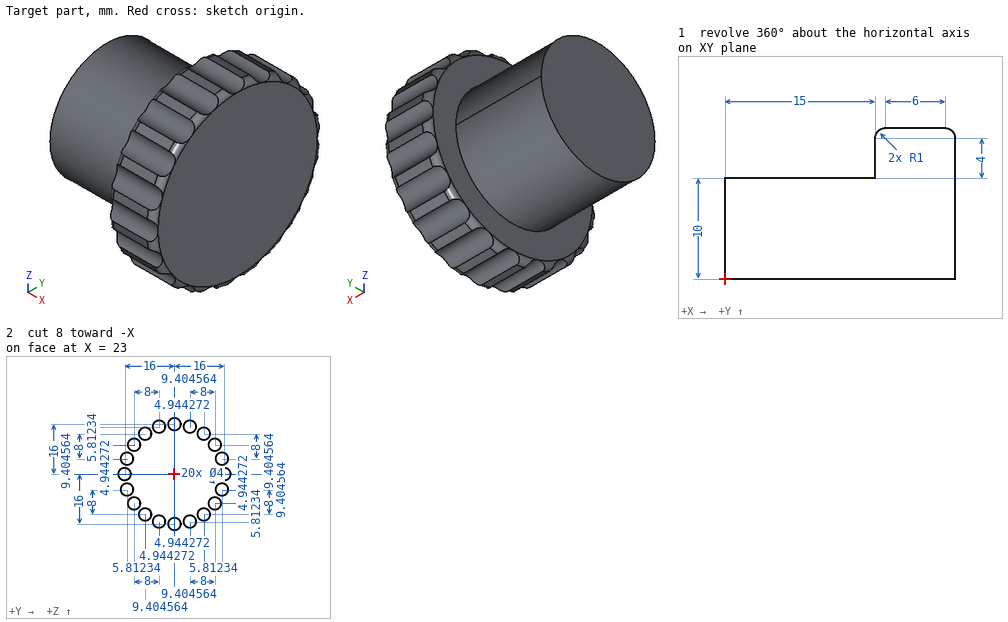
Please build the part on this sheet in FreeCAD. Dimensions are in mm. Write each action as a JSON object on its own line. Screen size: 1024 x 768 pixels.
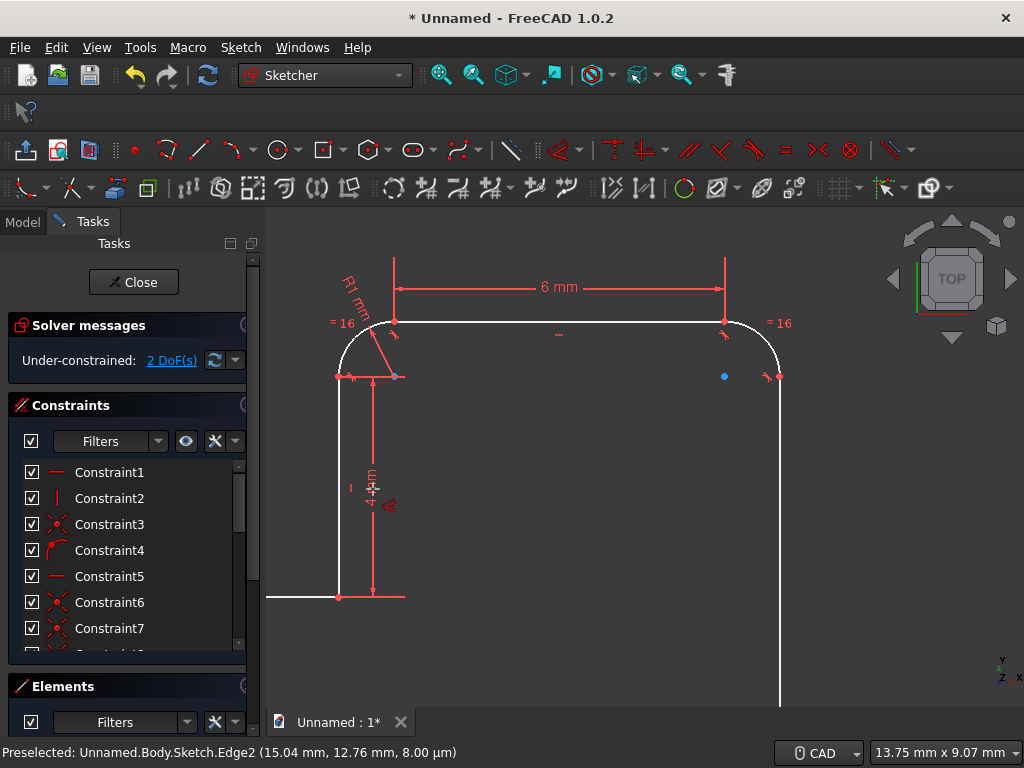
{"action": "scroll", "coordinate": [763, 337], "scroll_direction": "down", "scroll_amount": 6}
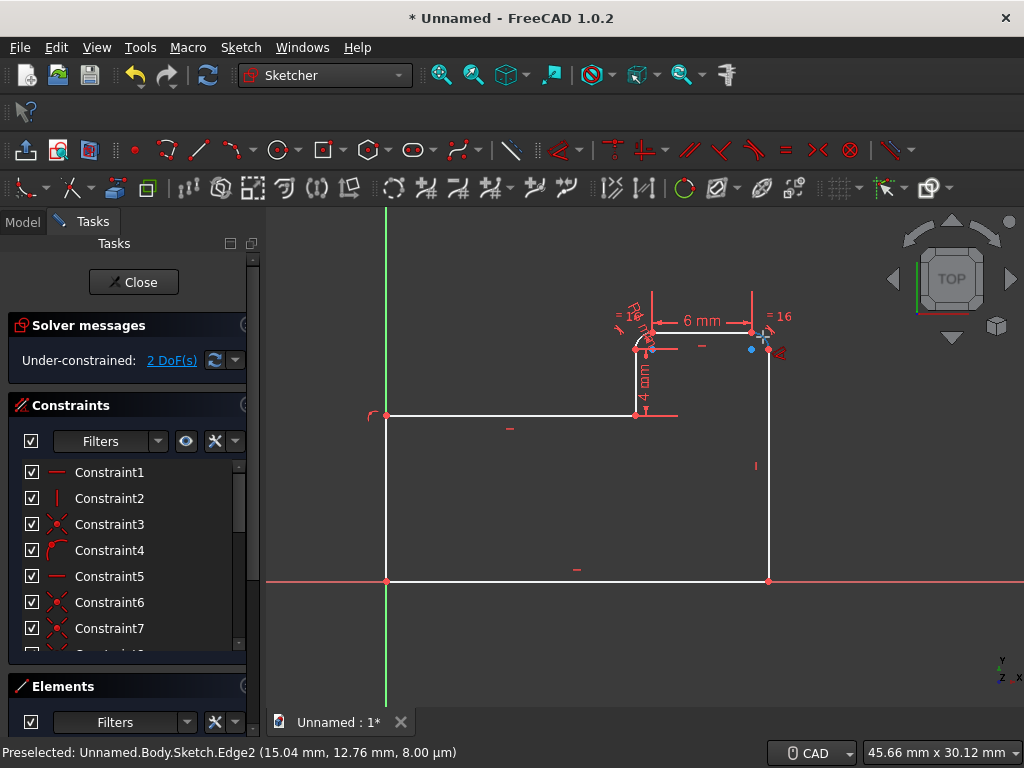
{"action": "left_click", "coordinate": [561, 416]}
{"action": "left_click", "coordinate": [511, 382]}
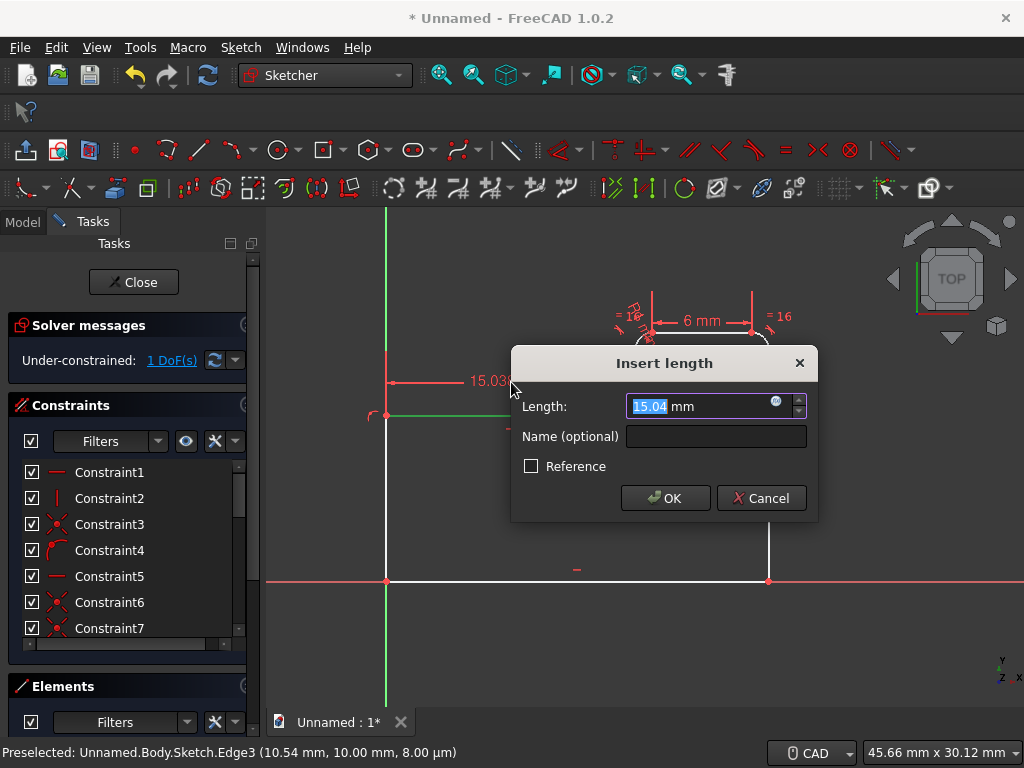
{"action": "type", "text": "15"}
{"action": "key", "text": "Return"}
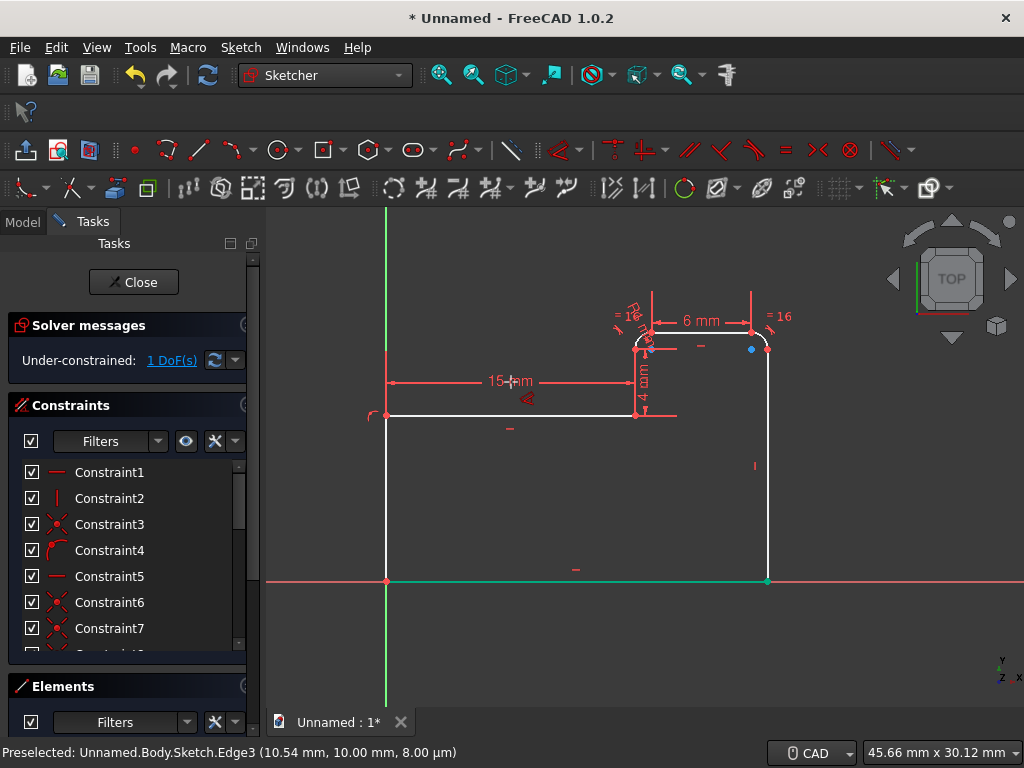
{"action": "left_click", "coordinate": [386, 465]}
{"action": "left_click", "coordinate": [352, 499]}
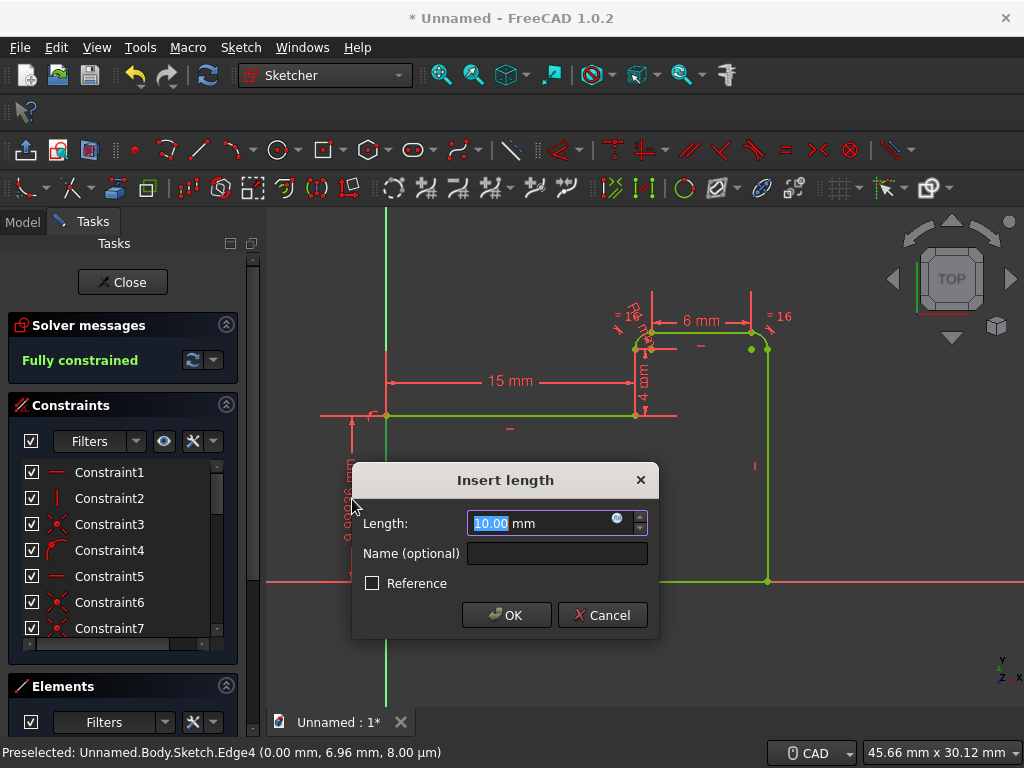
{"action": "type", "text": "10"}
{"action": "key", "text": "Return"}
{"action": "key", "text": "Escape"}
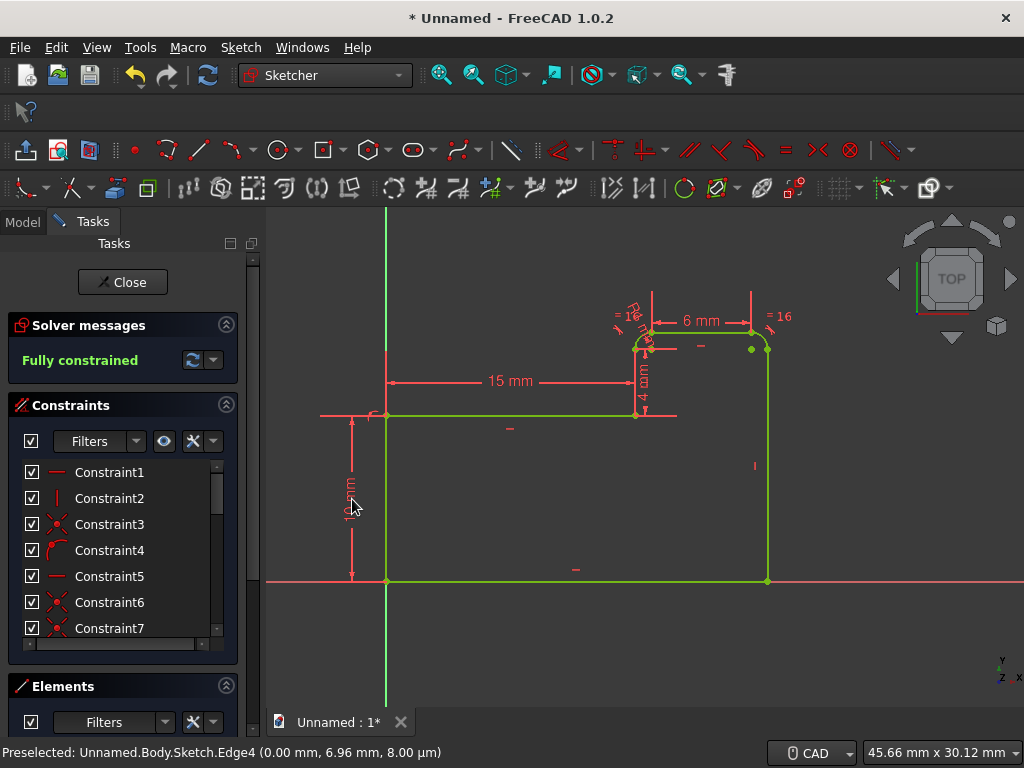
{"action": "left_click", "coordinate": [123, 282]}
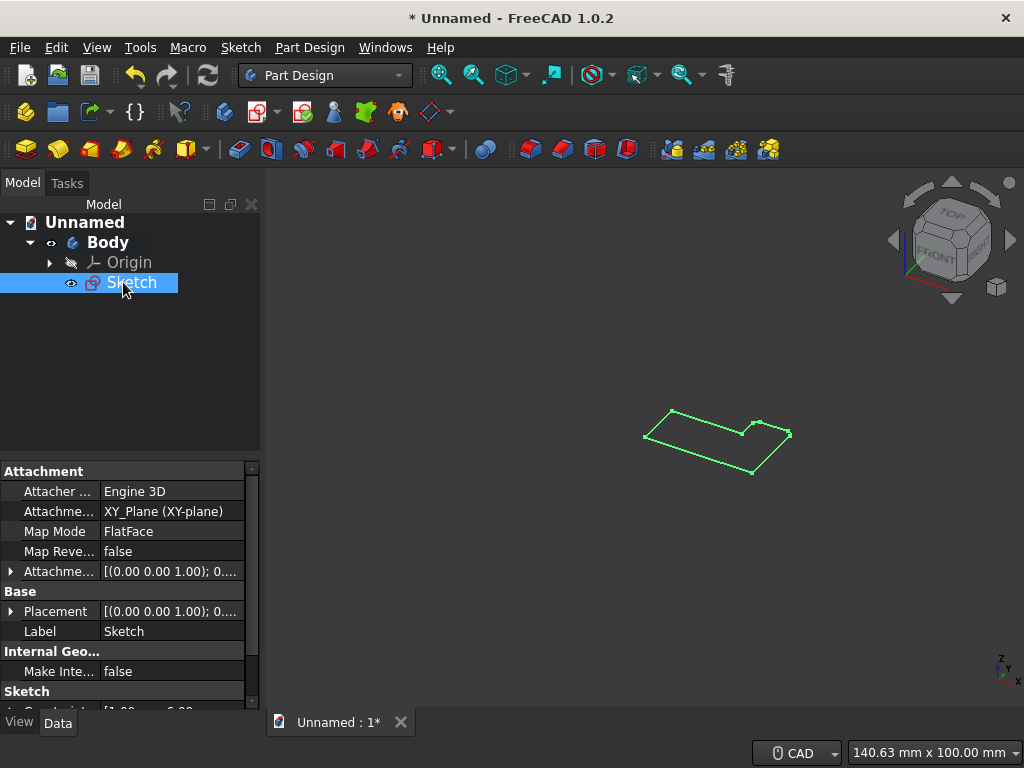
{"action": "left_click", "coordinate": [58, 150]}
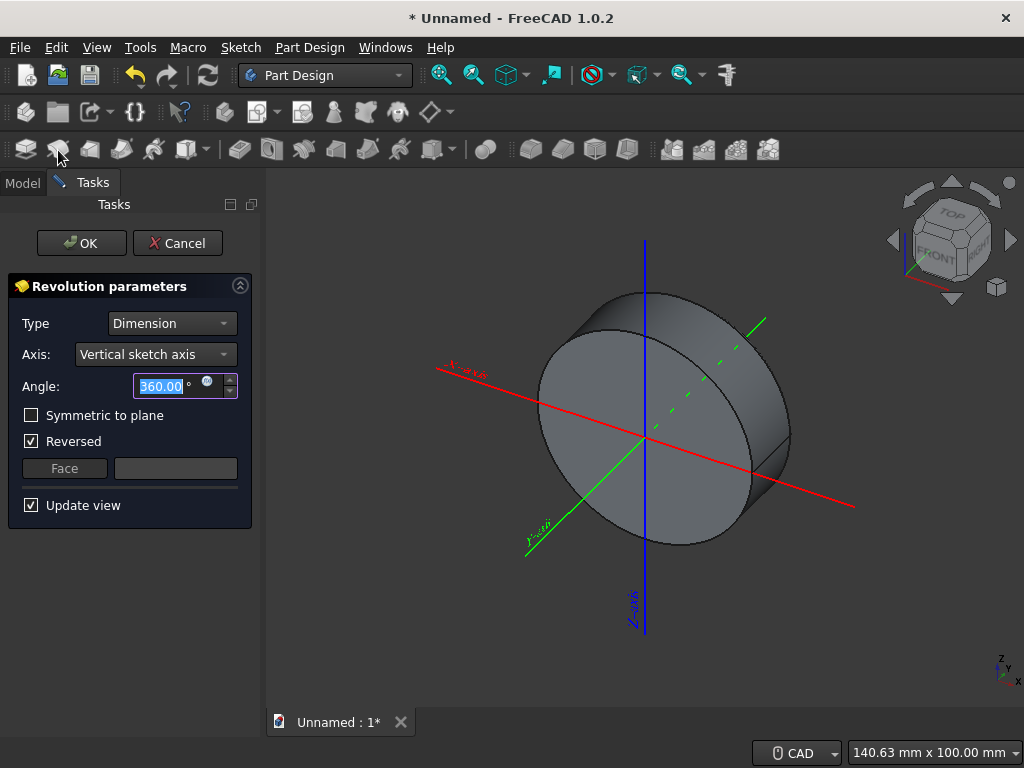
{"action": "left_click", "coordinate": [156, 354]}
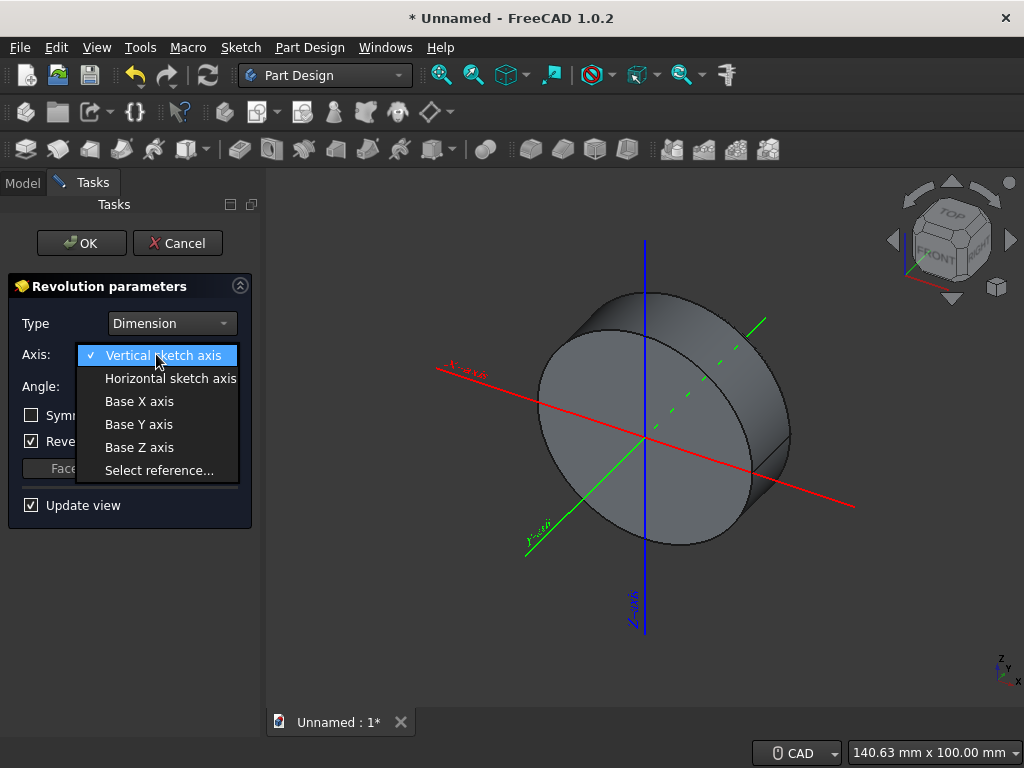
{"action": "left_click", "coordinate": [156, 378]}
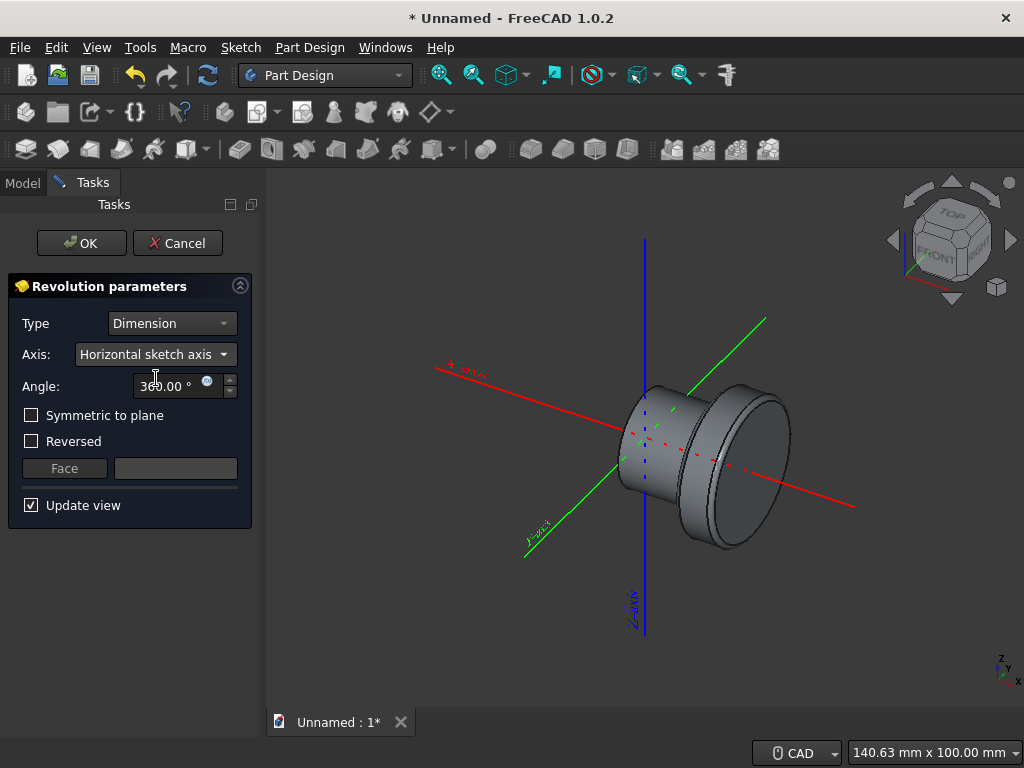
{"action": "left_click", "coordinate": [82, 243]}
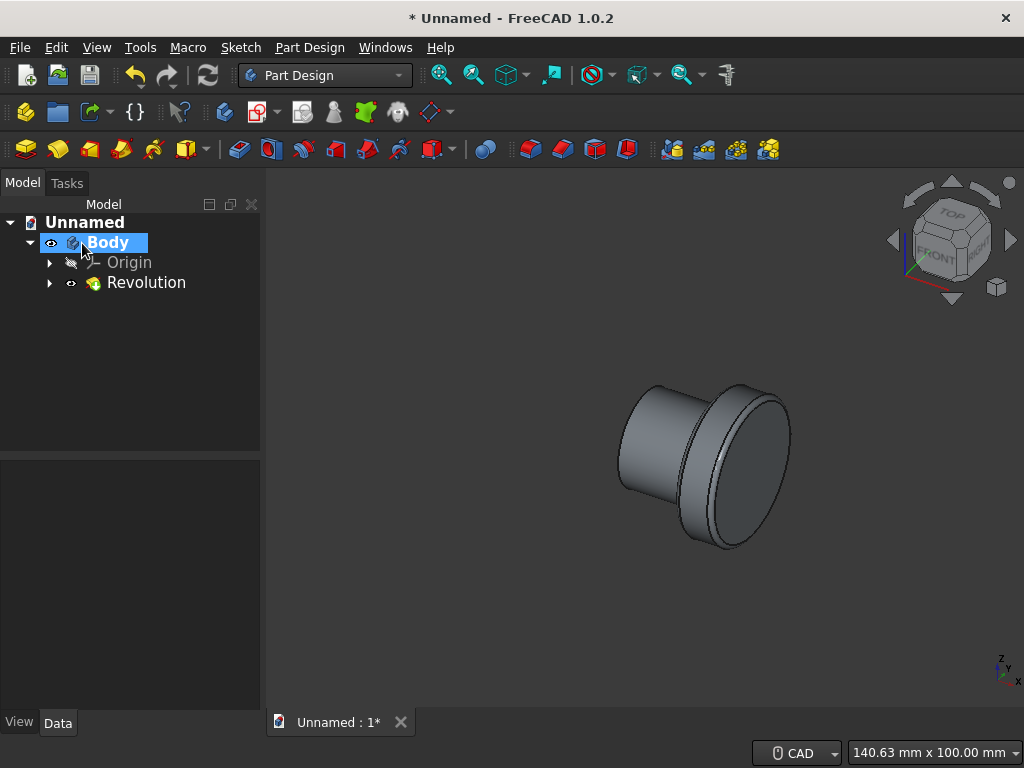
{"action": "left_click", "coordinate": [752, 472]}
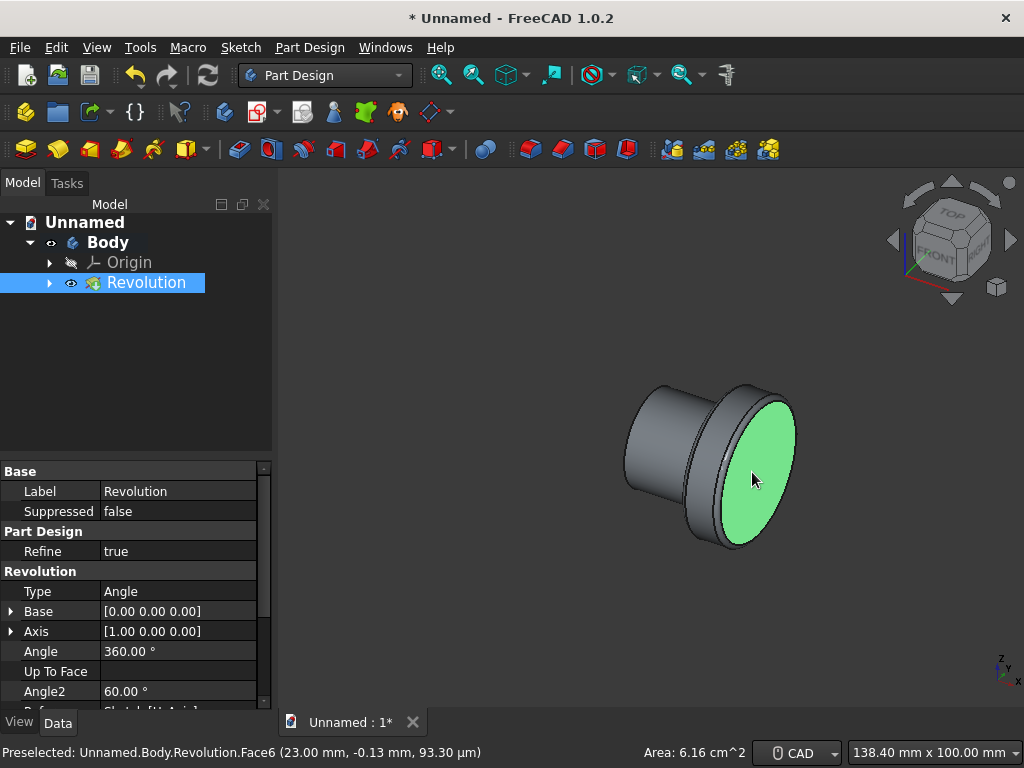
{"action": "left_click", "coordinate": [258, 112]}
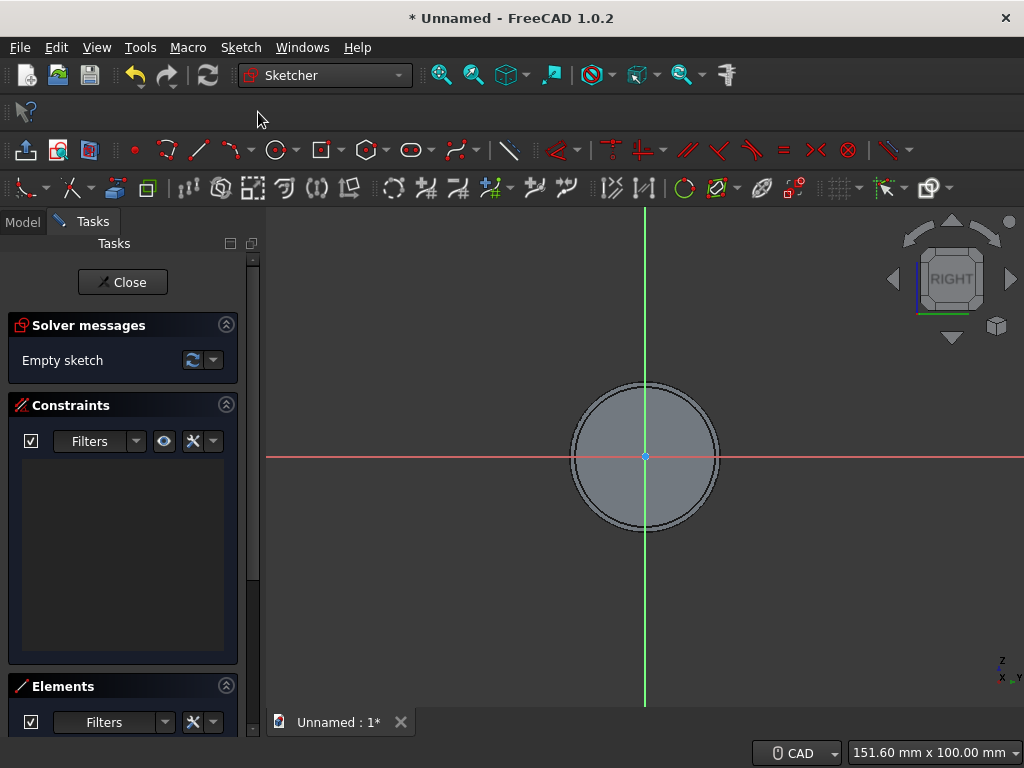
{"action": "scroll", "coordinate": [728, 457], "scroll_direction": "up", "scroll_amount": 3}